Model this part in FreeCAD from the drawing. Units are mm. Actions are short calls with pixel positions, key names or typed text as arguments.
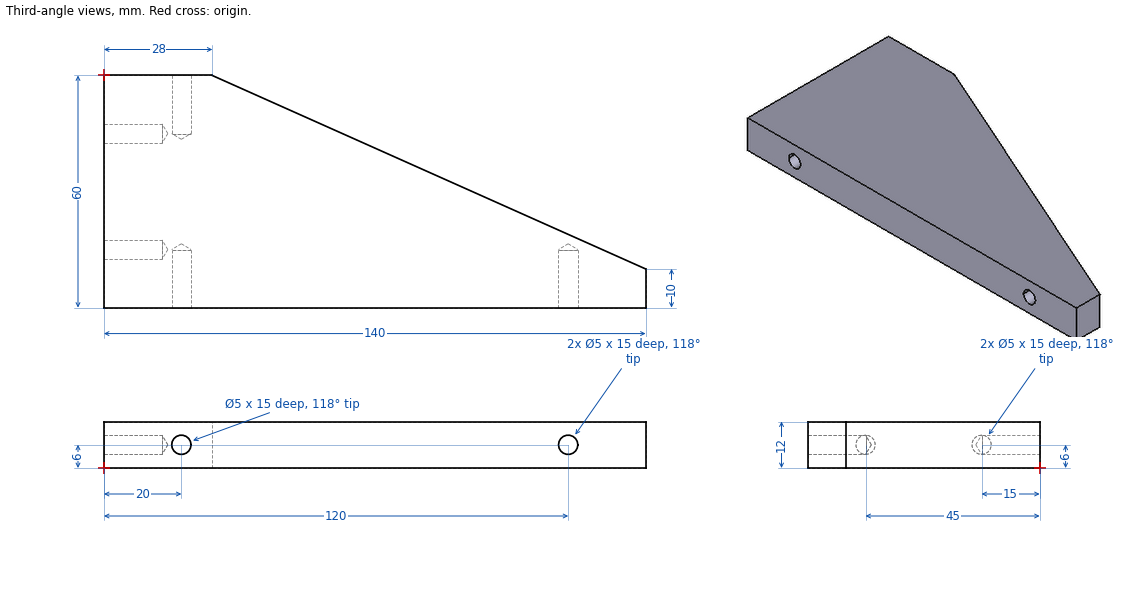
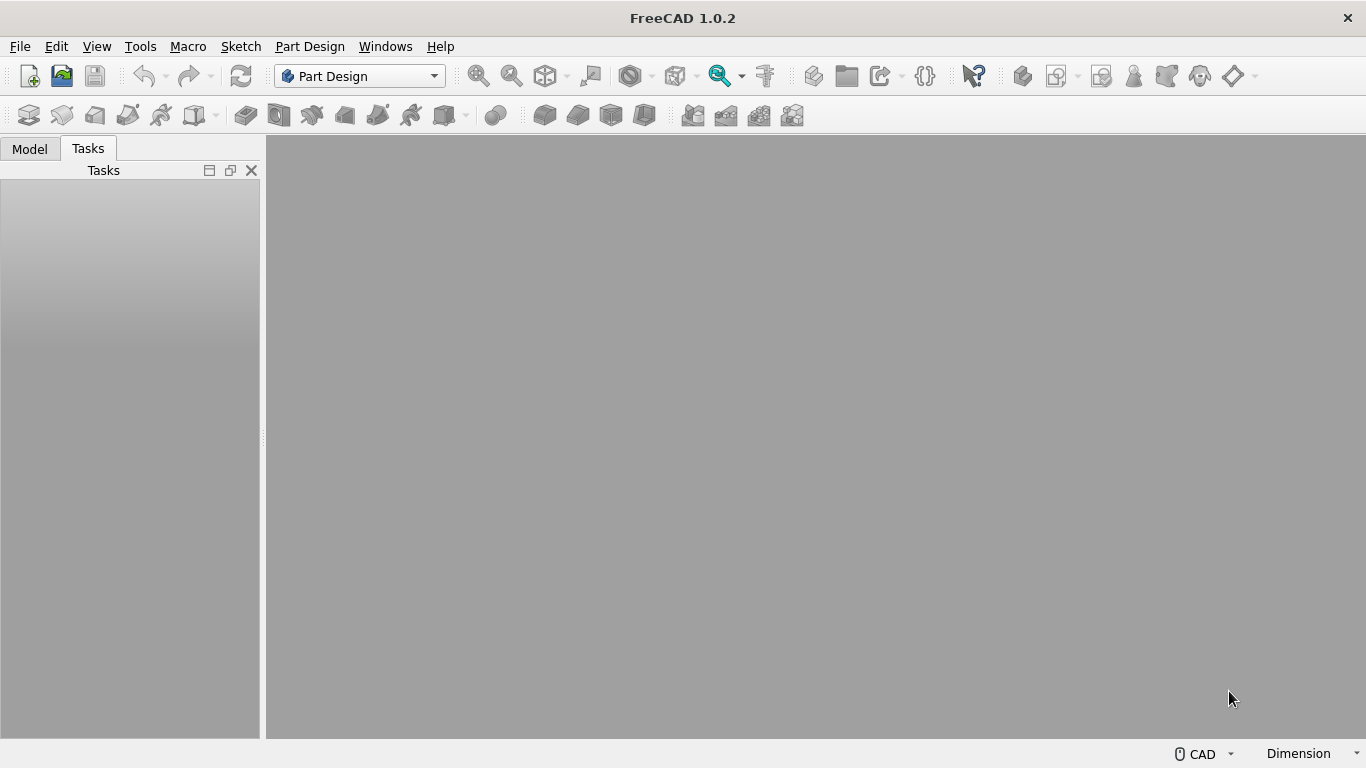
click(29, 76)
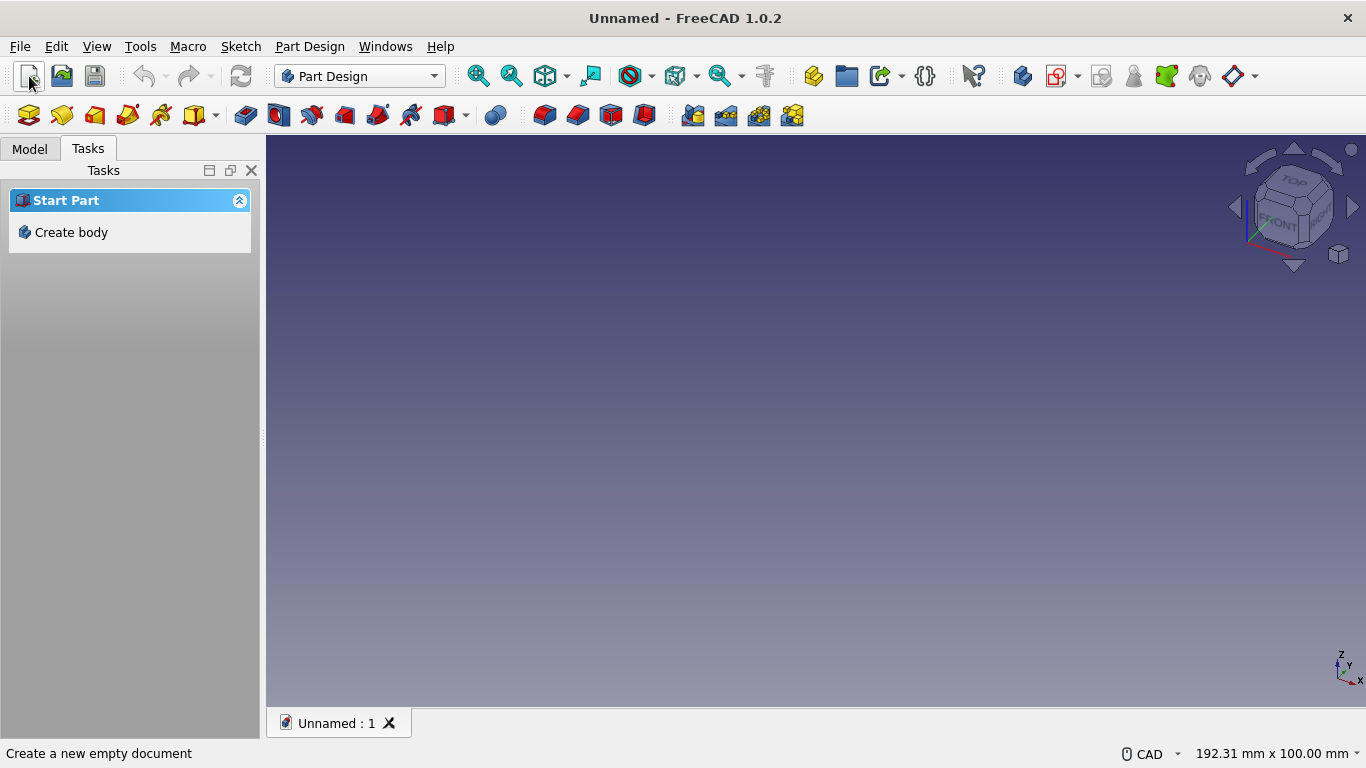
click(1056, 76)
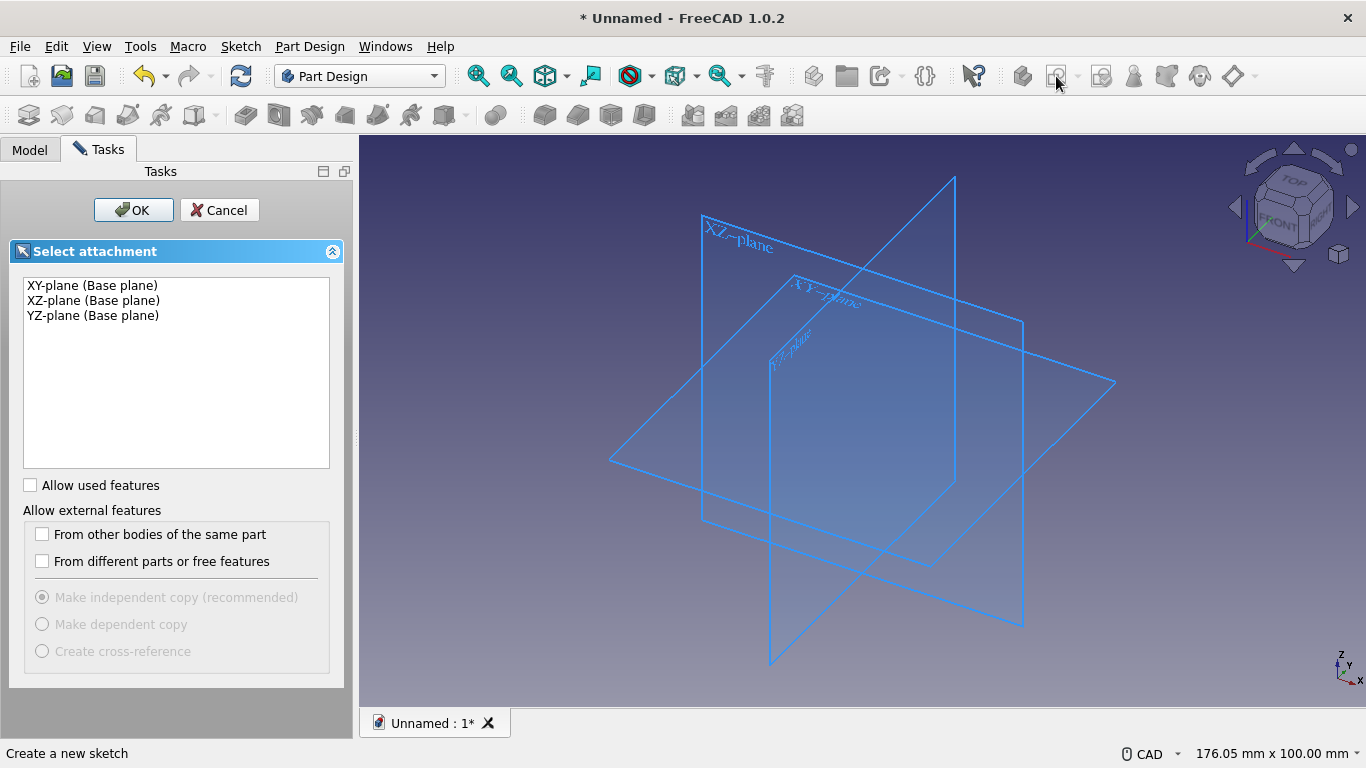
click(84, 286)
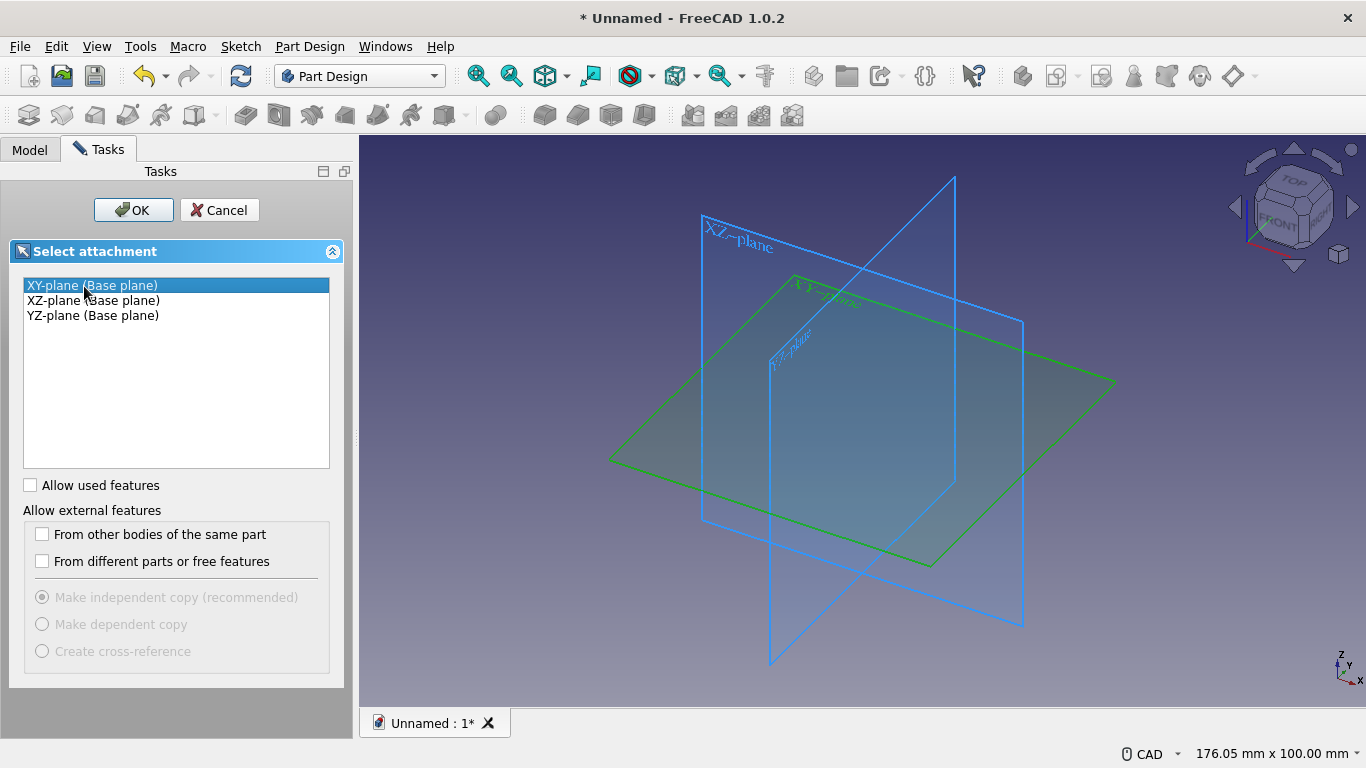
click(134, 210)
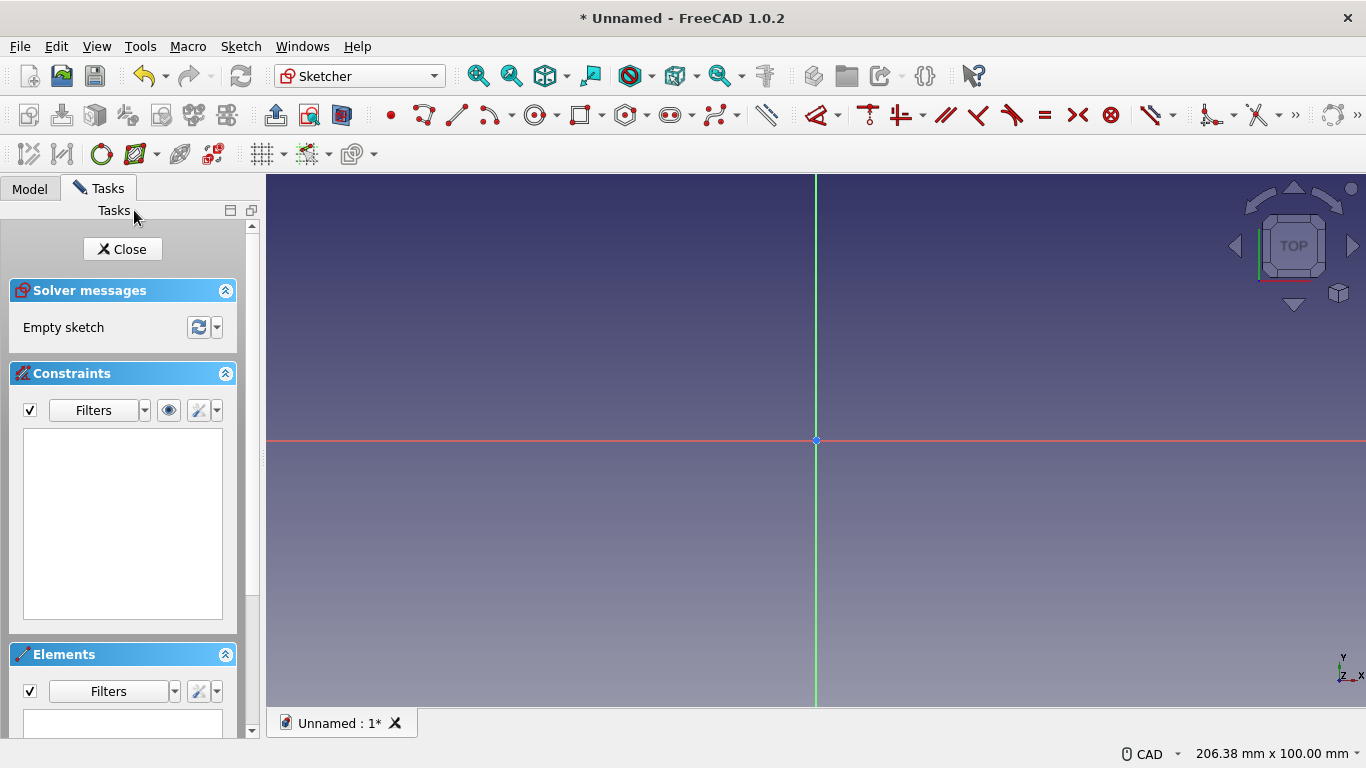
scroll(294, 202, down, 2)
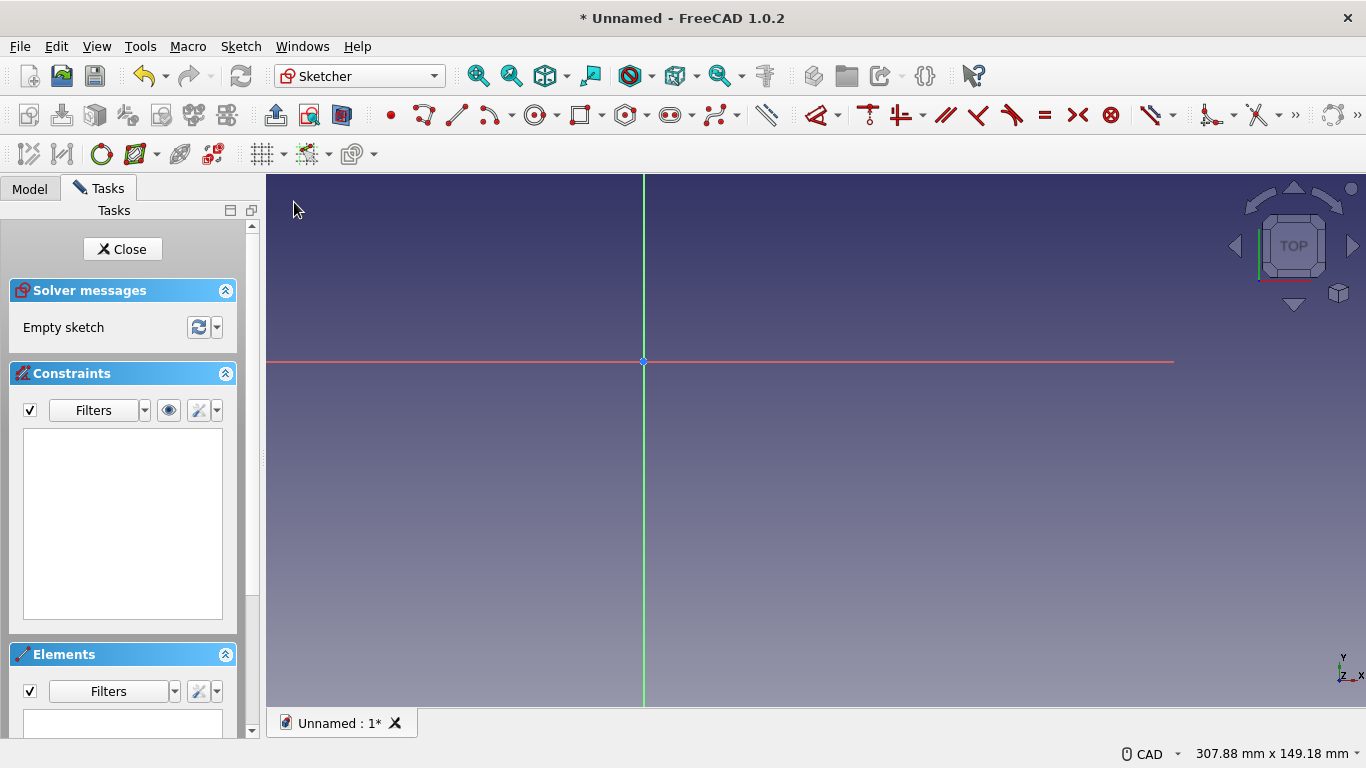
click(424, 116)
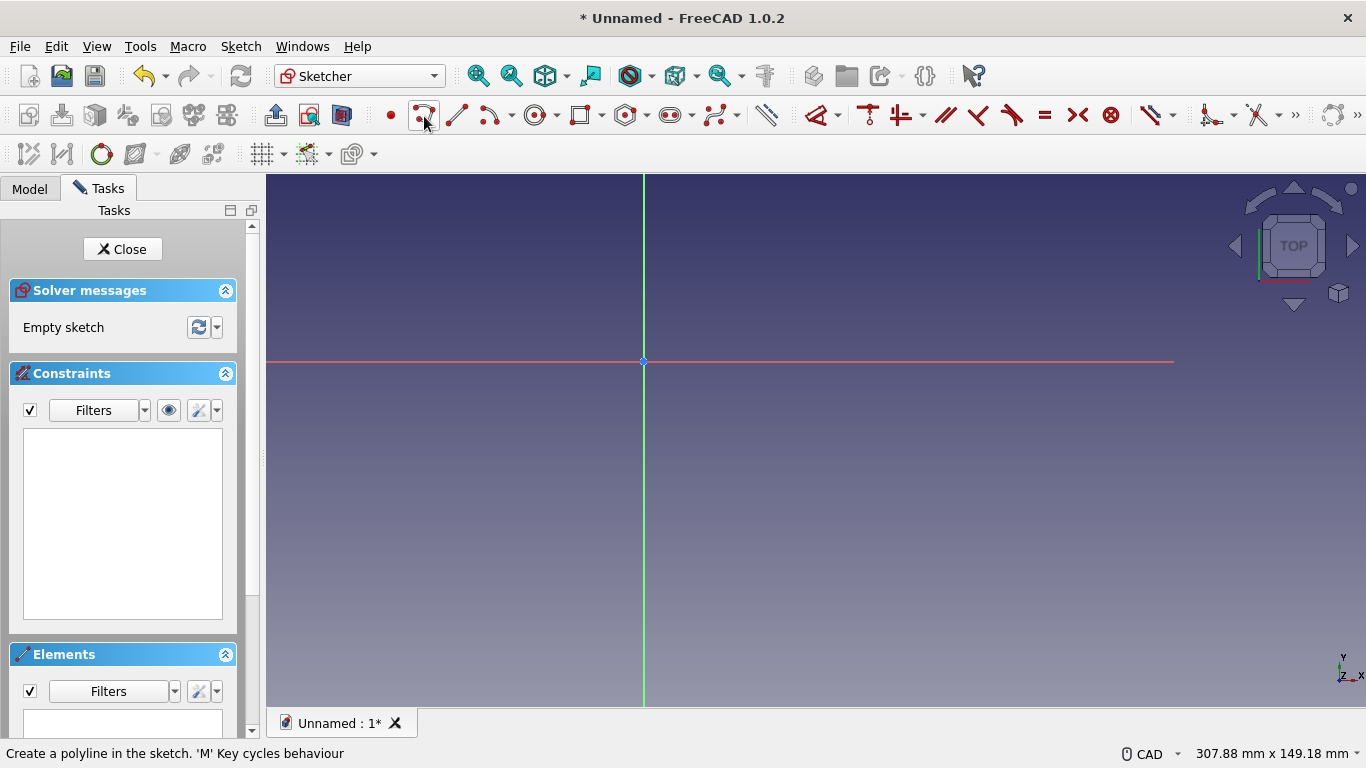
click(644, 362)
click(653, 576)
click(1144, 576)
click(1144, 541)
click(744, 371)
click(644, 362)
key(Escape)
key(Escape)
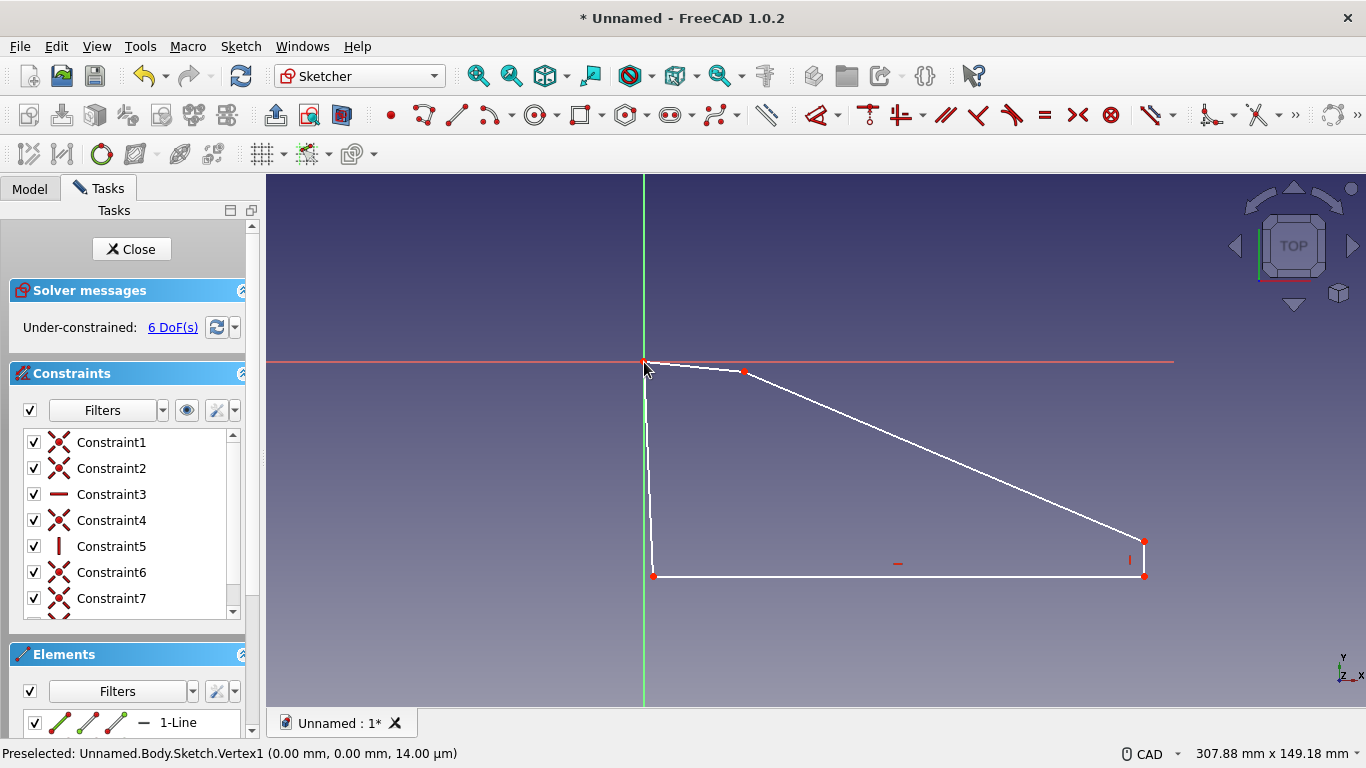
click(647, 426)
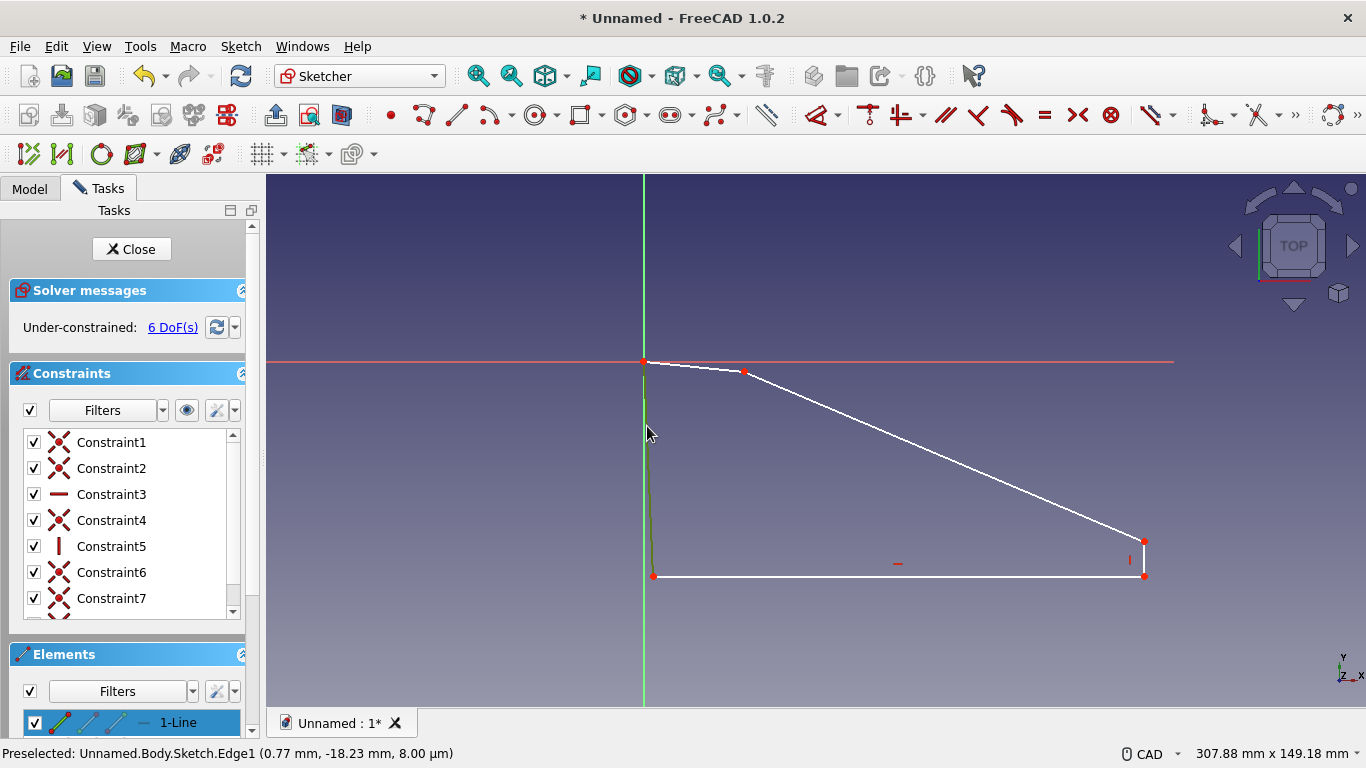
click(922, 116)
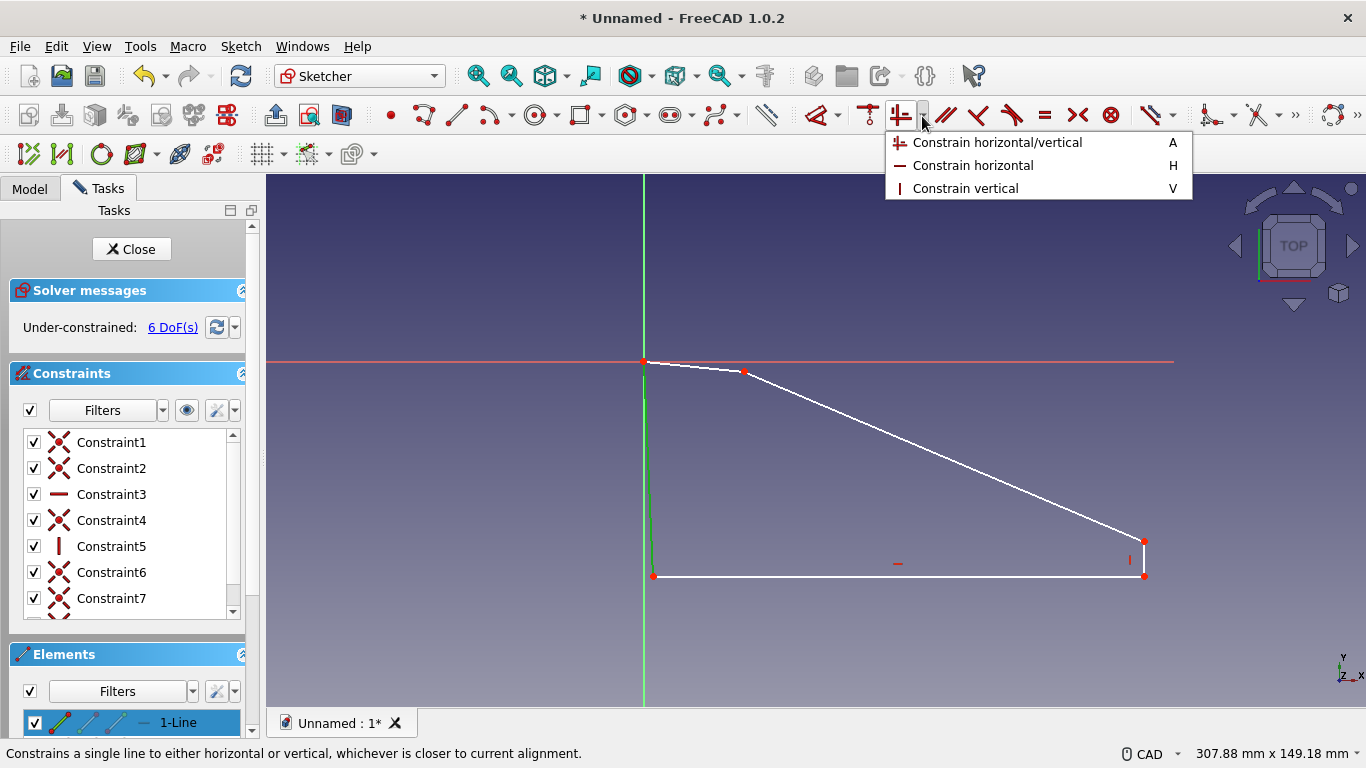
click(1039, 188)